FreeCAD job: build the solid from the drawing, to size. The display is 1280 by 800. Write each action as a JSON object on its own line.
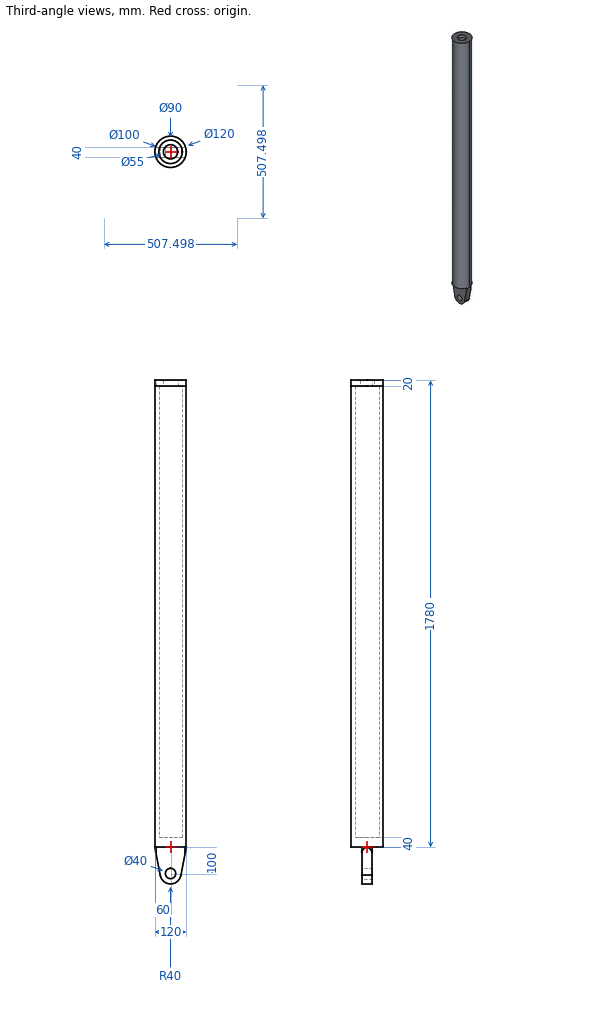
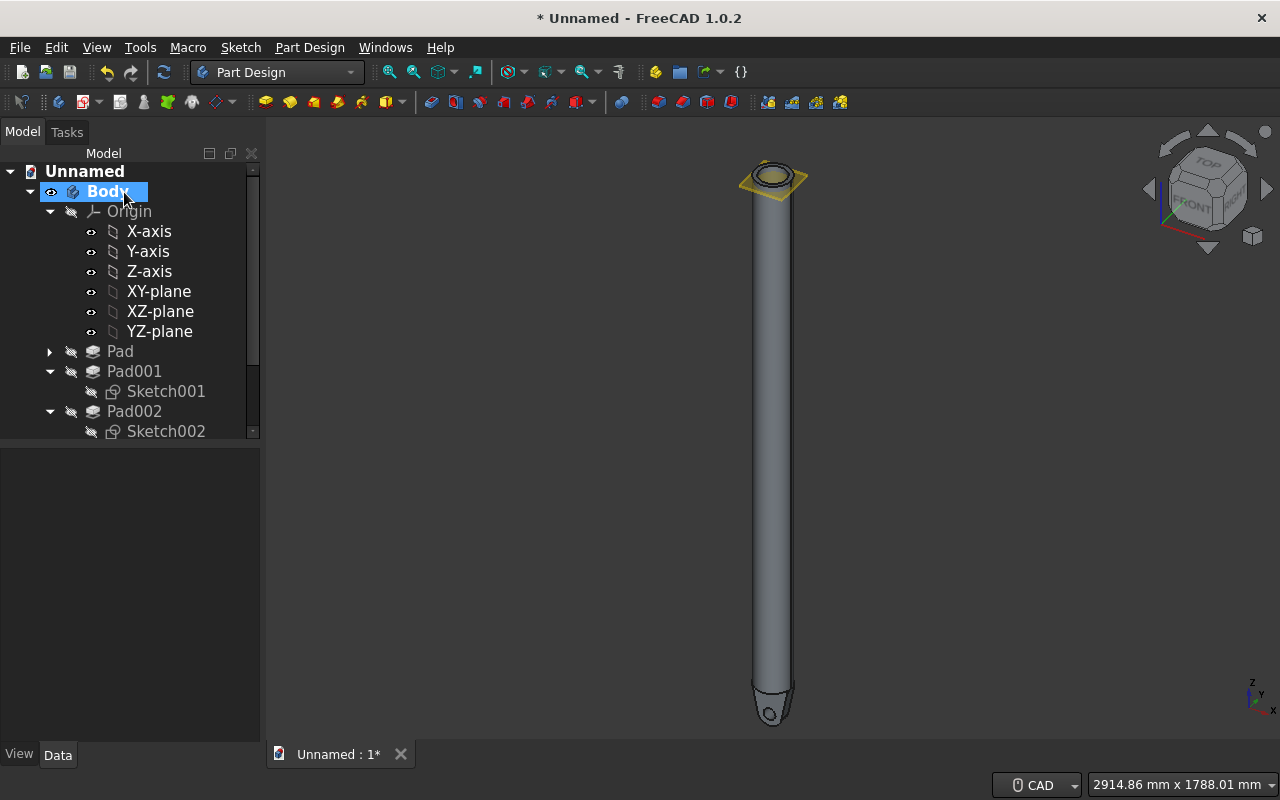
{"action": "scroll", "coordinate": [100, 307], "scroll_direction": "down", "scroll_amount": 3}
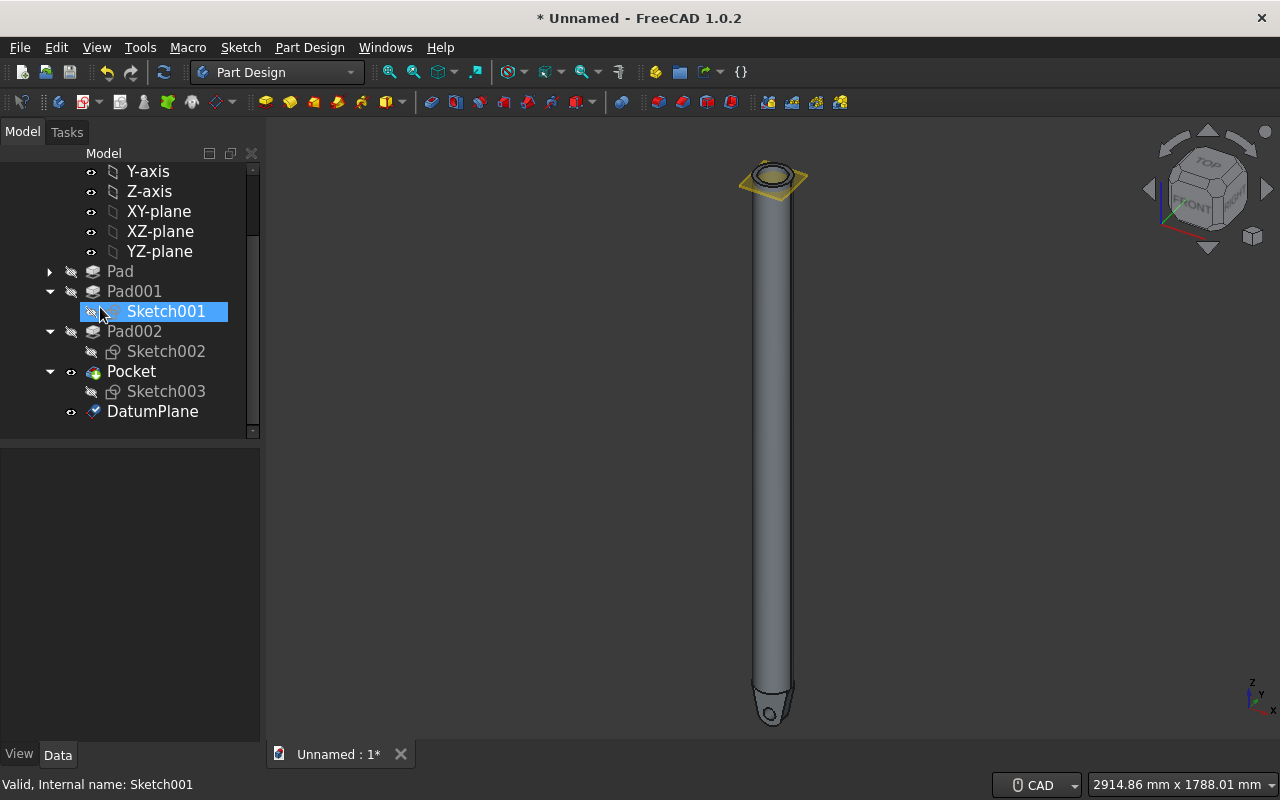
{"action": "left_click", "coordinate": [116, 412]}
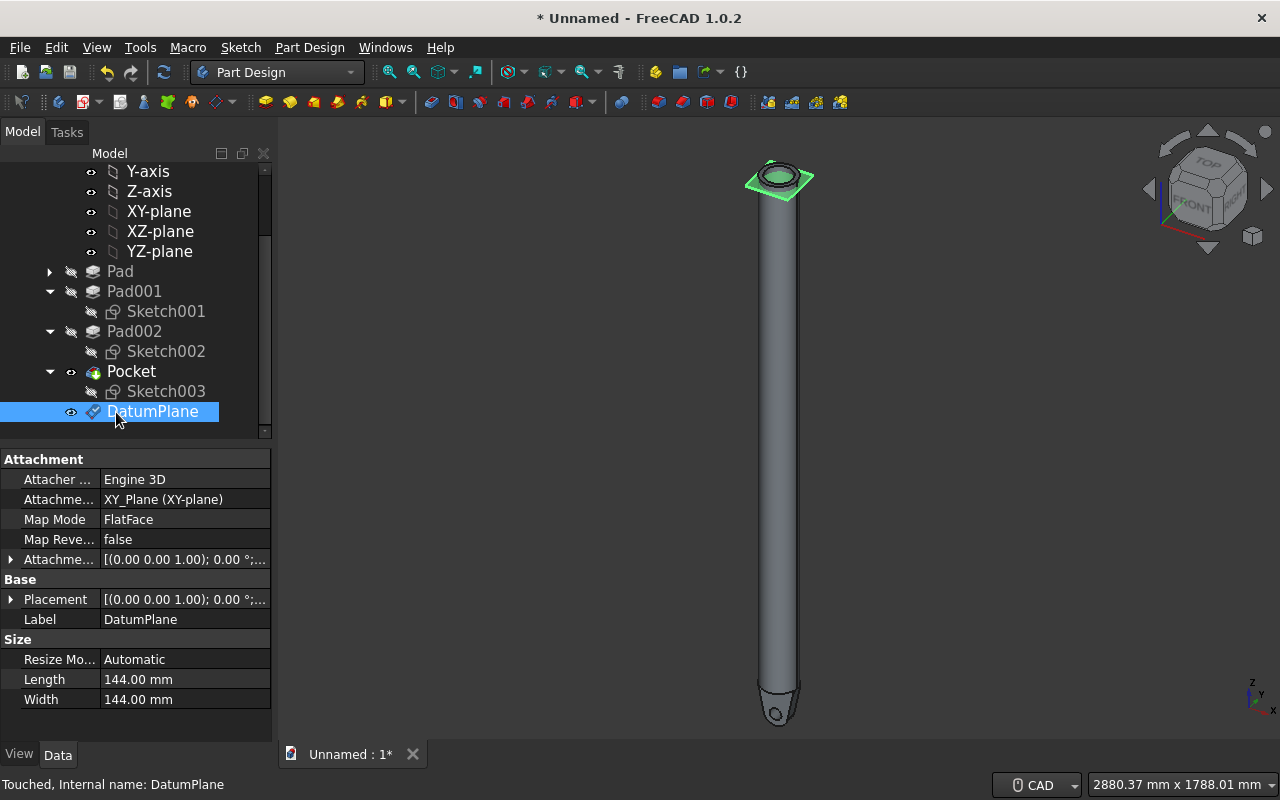
{"action": "left_click", "coordinate": [84, 102]}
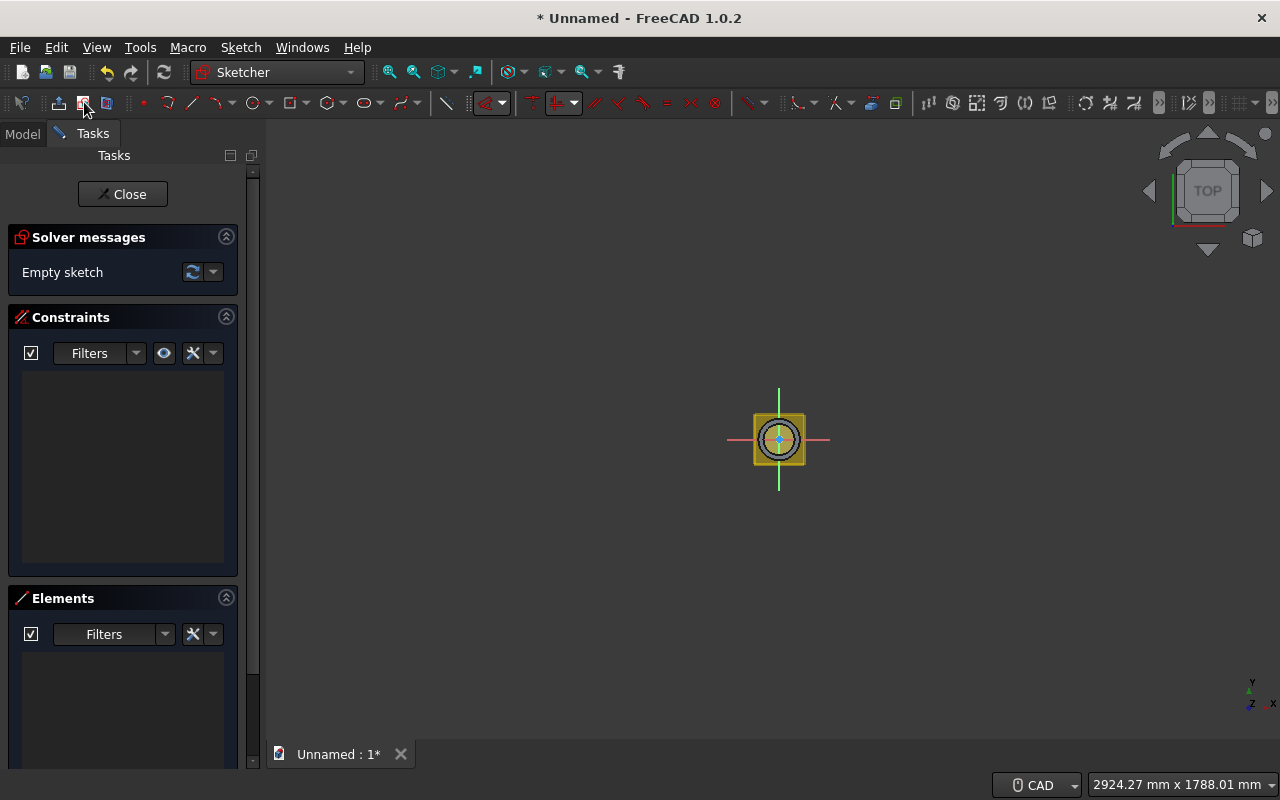
{"action": "key", "text": "q s"}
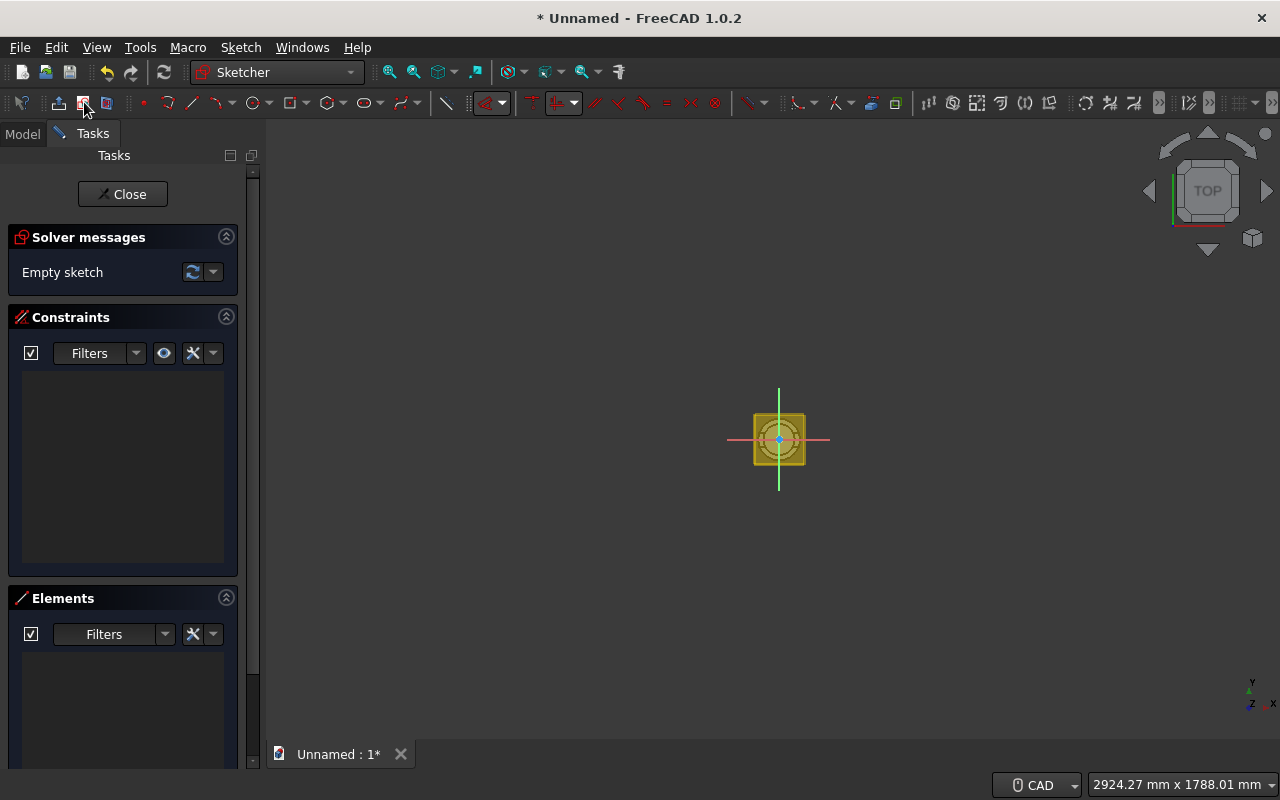
{"action": "scroll", "coordinate": [788, 441], "scroll_direction": "up", "scroll_amount": 11}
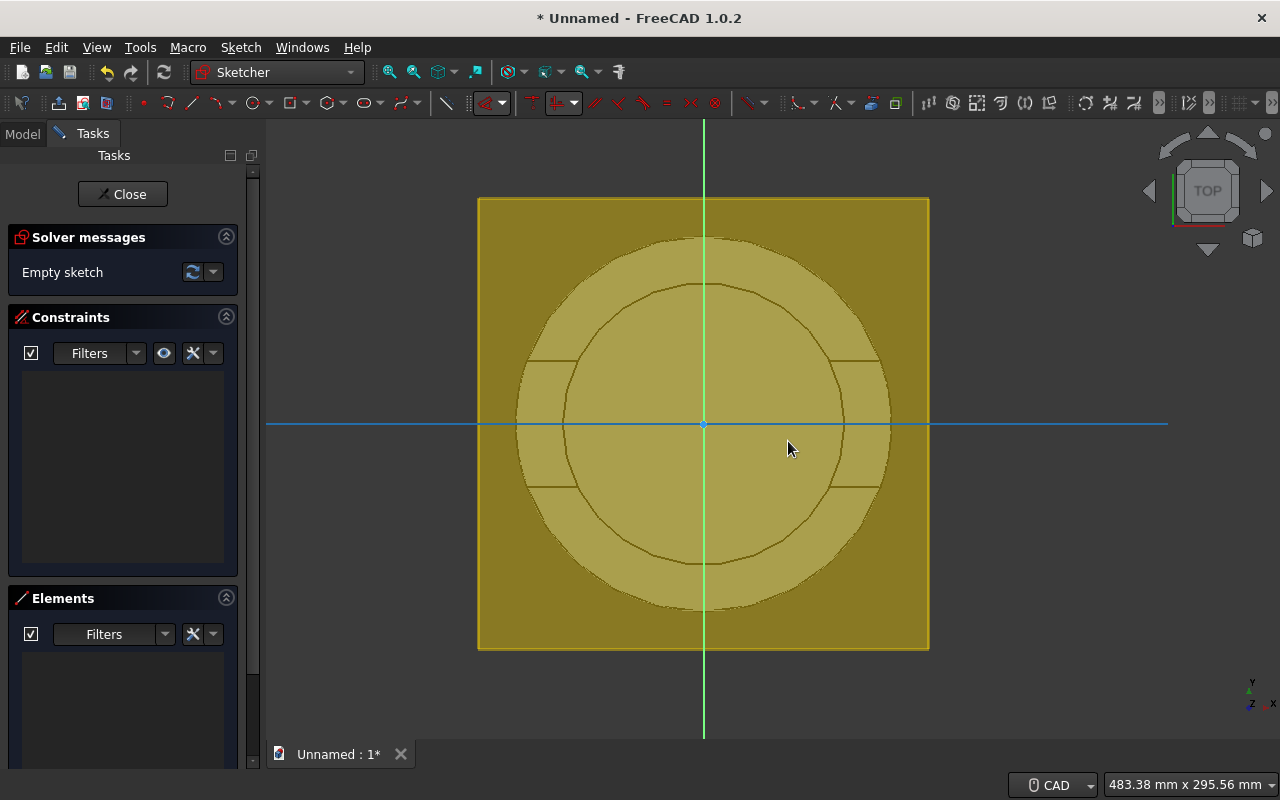
{"action": "key", "text": "g c"}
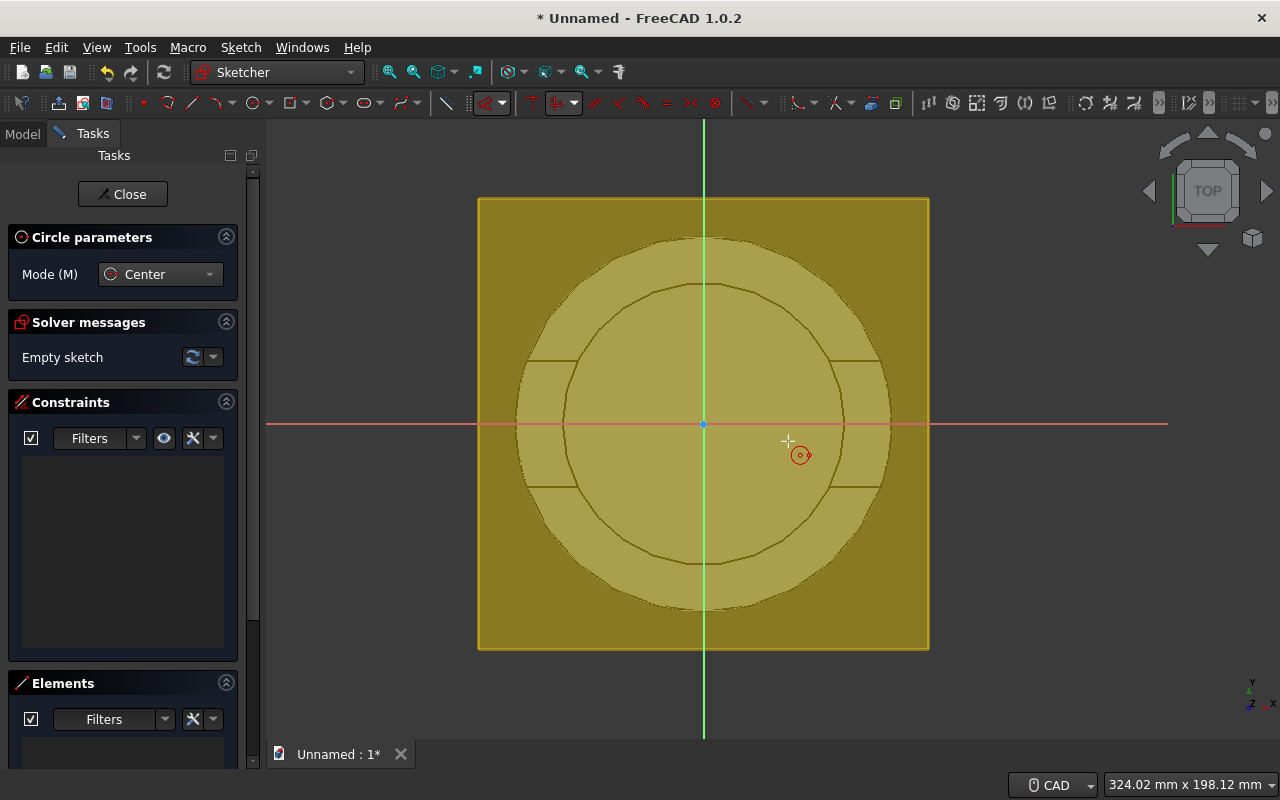
{"action": "left_click", "coordinate": [704, 424]}
{"action": "mouse_move", "coordinate": [836, 291]}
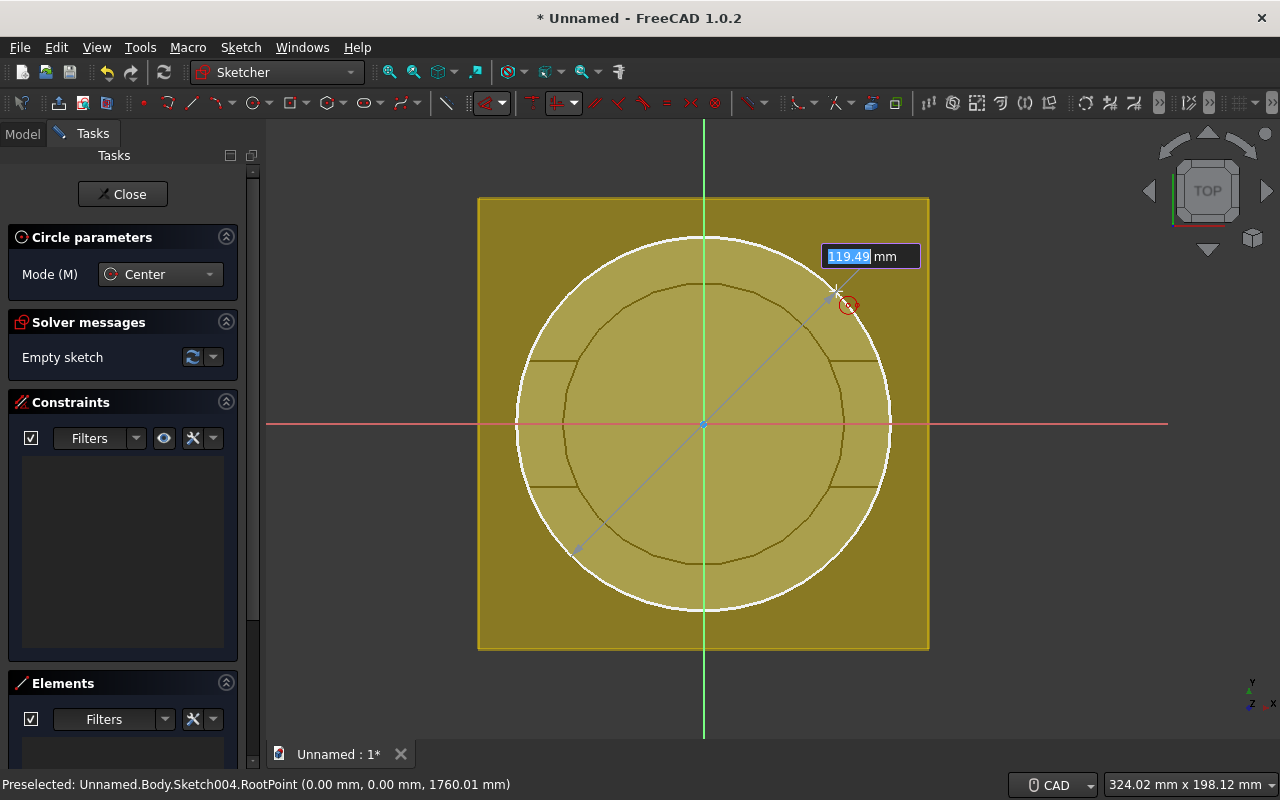
{"action": "type", "text": "120"}
{"action": "key", "text": "Return"}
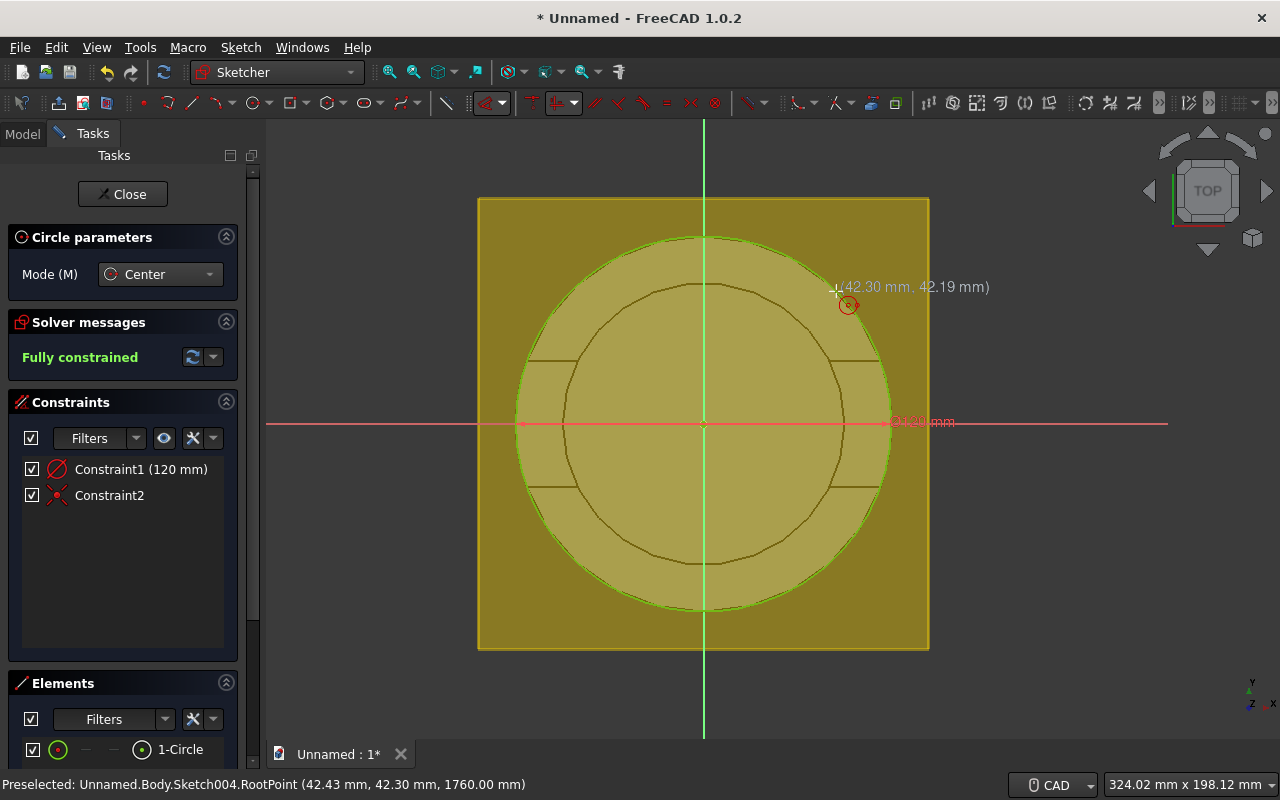
{"action": "left_click", "coordinate": [704, 424]}
{"action": "mouse_move", "coordinate": [764, 363]}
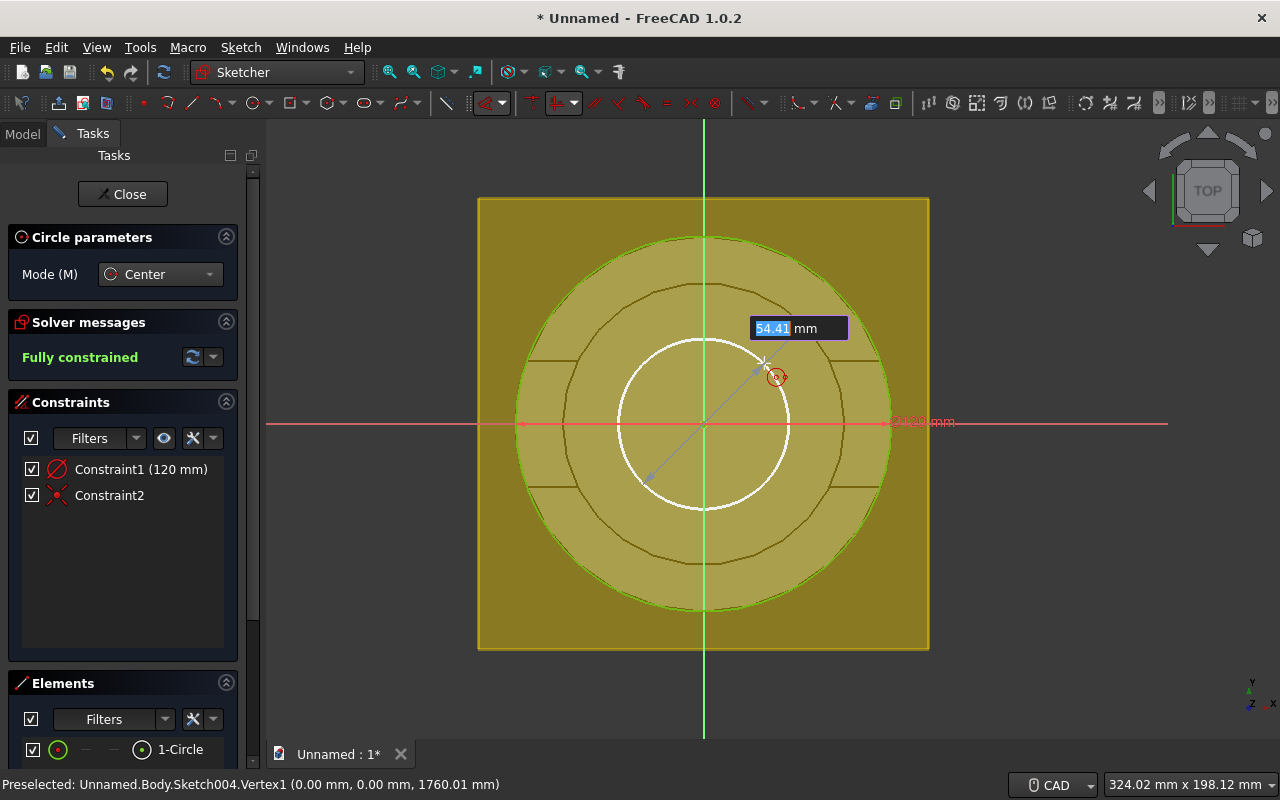
{"action": "type", "text": "55"}
{"action": "key", "text": "Return"}
{"action": "key", "text": "Escape"}